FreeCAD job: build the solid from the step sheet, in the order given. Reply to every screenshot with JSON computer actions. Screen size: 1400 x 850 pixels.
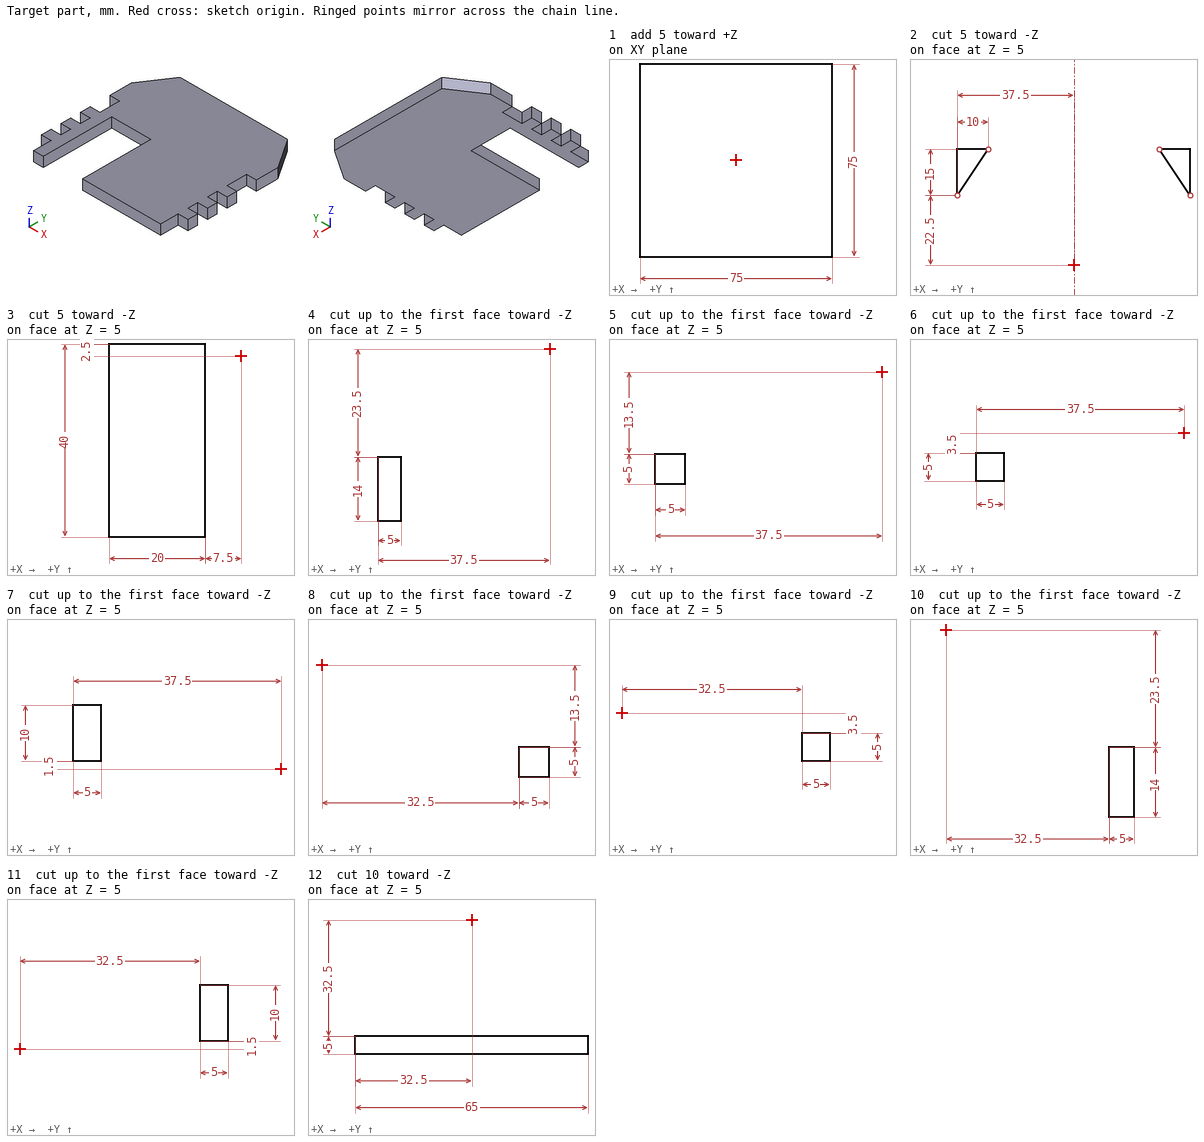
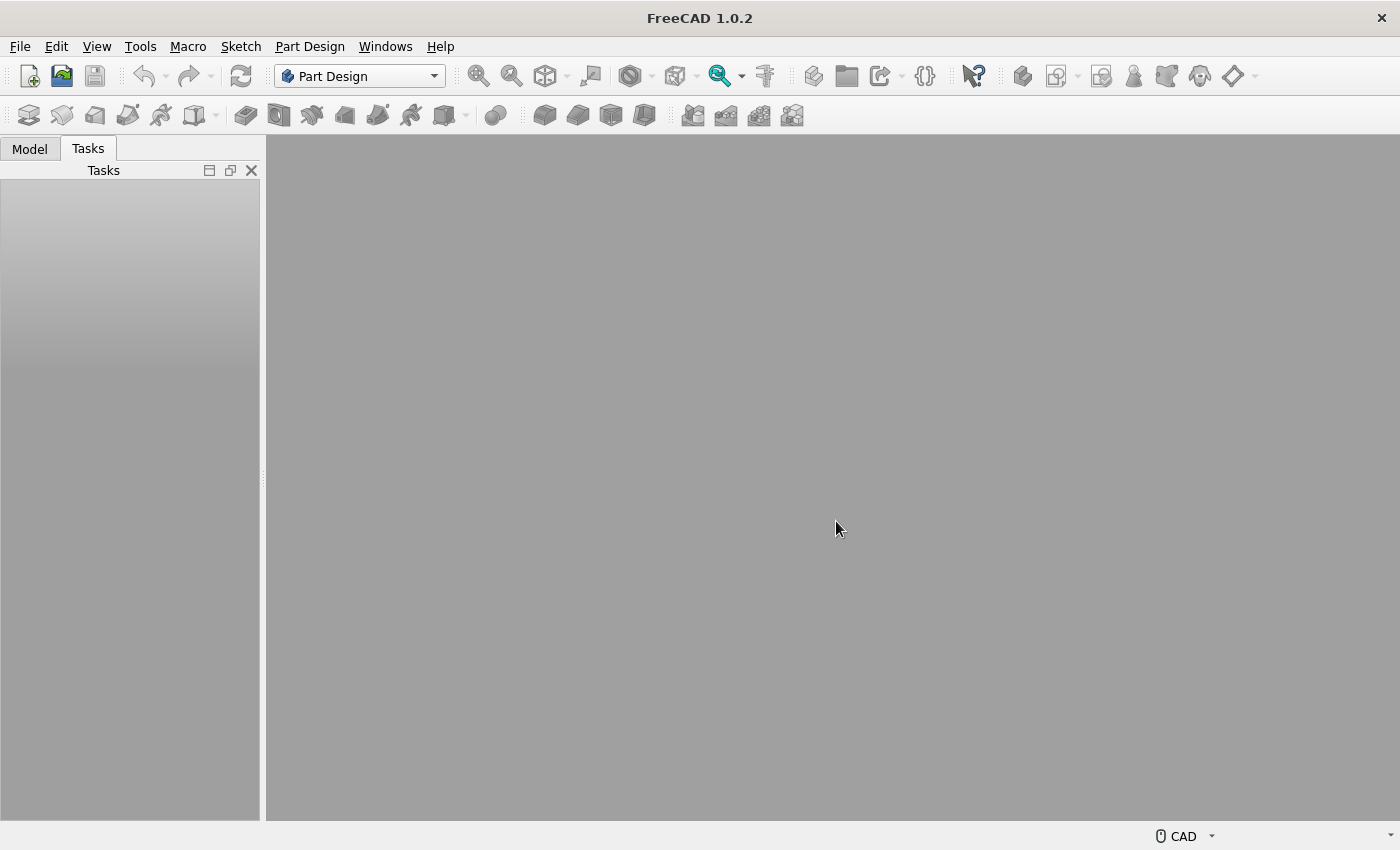
{"action": "left_click", "coordinate": [29, 76]}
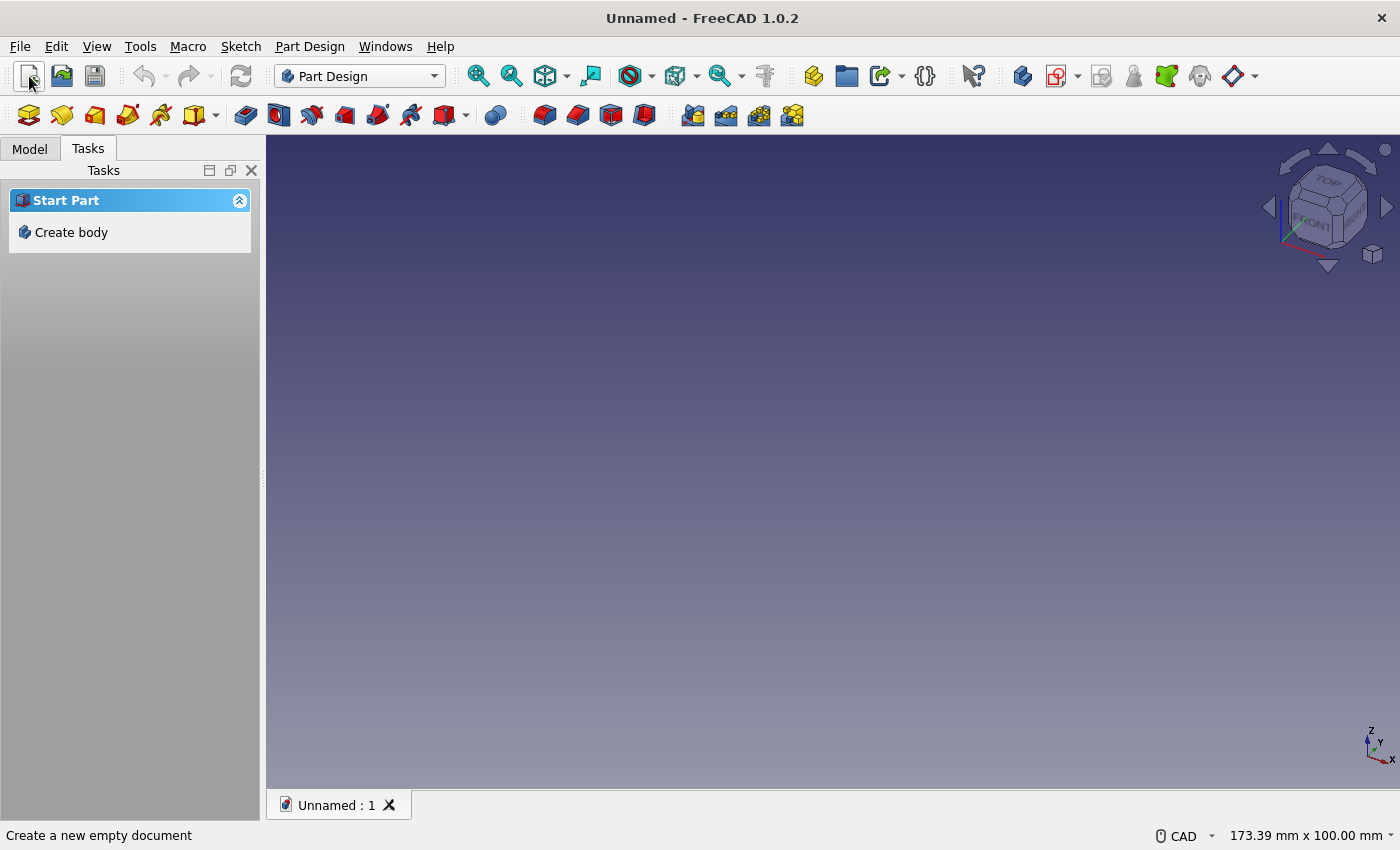
{"action": "left_click", "coordinate": [1056, 76]}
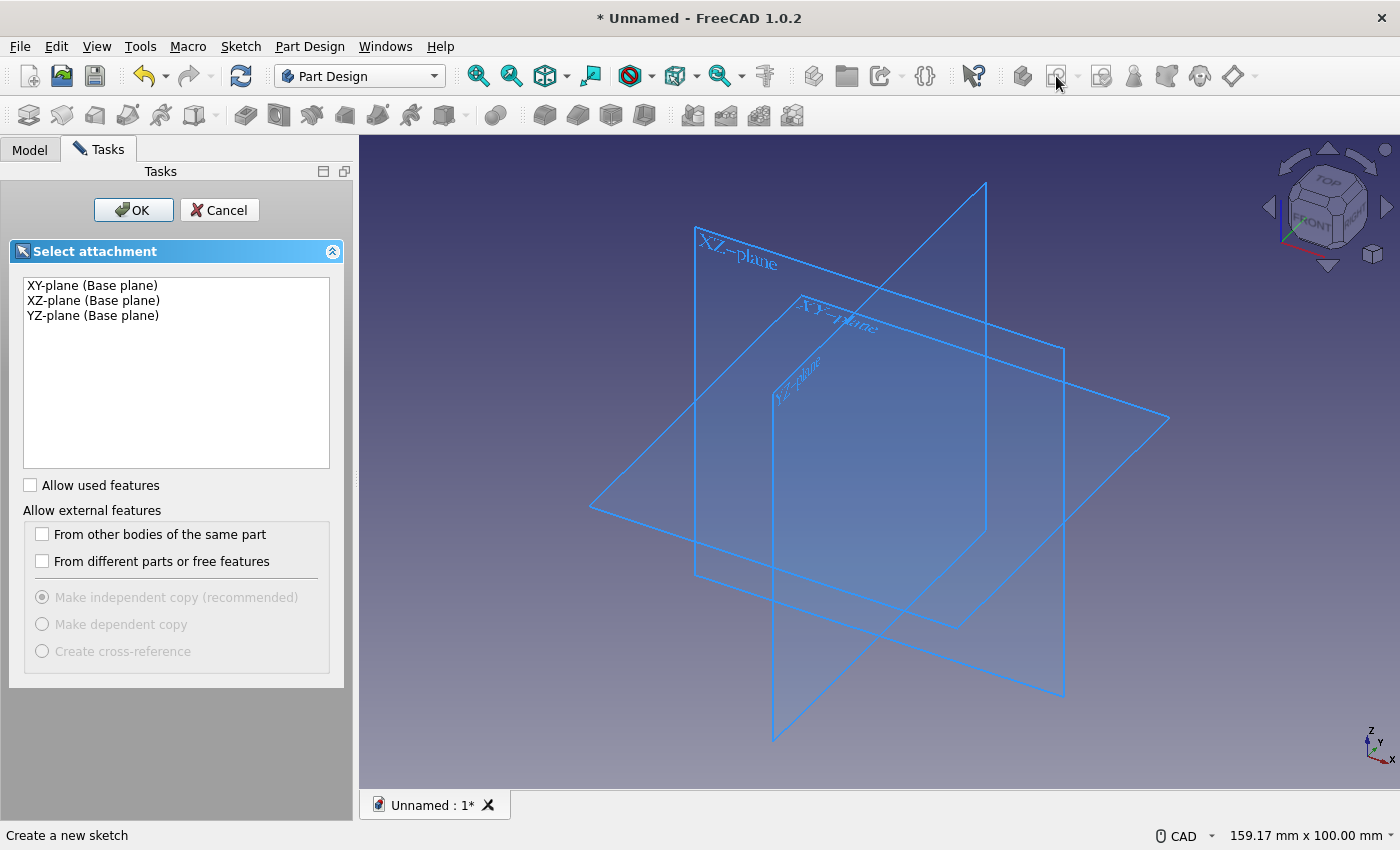
{"action": "left_click", "coordinate": [84, 286]}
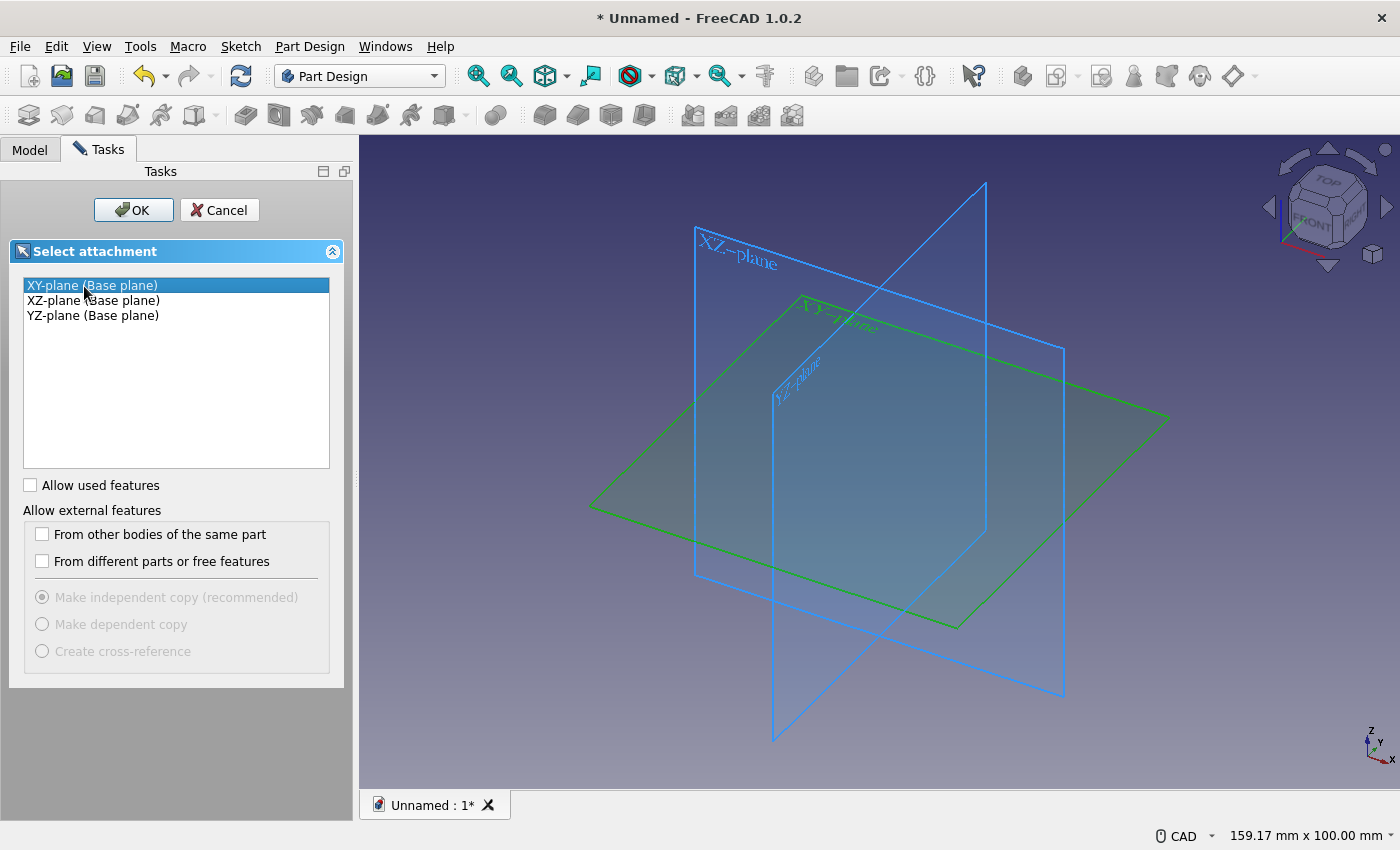
{"action": "left_click", "coordinate": [134, 210]}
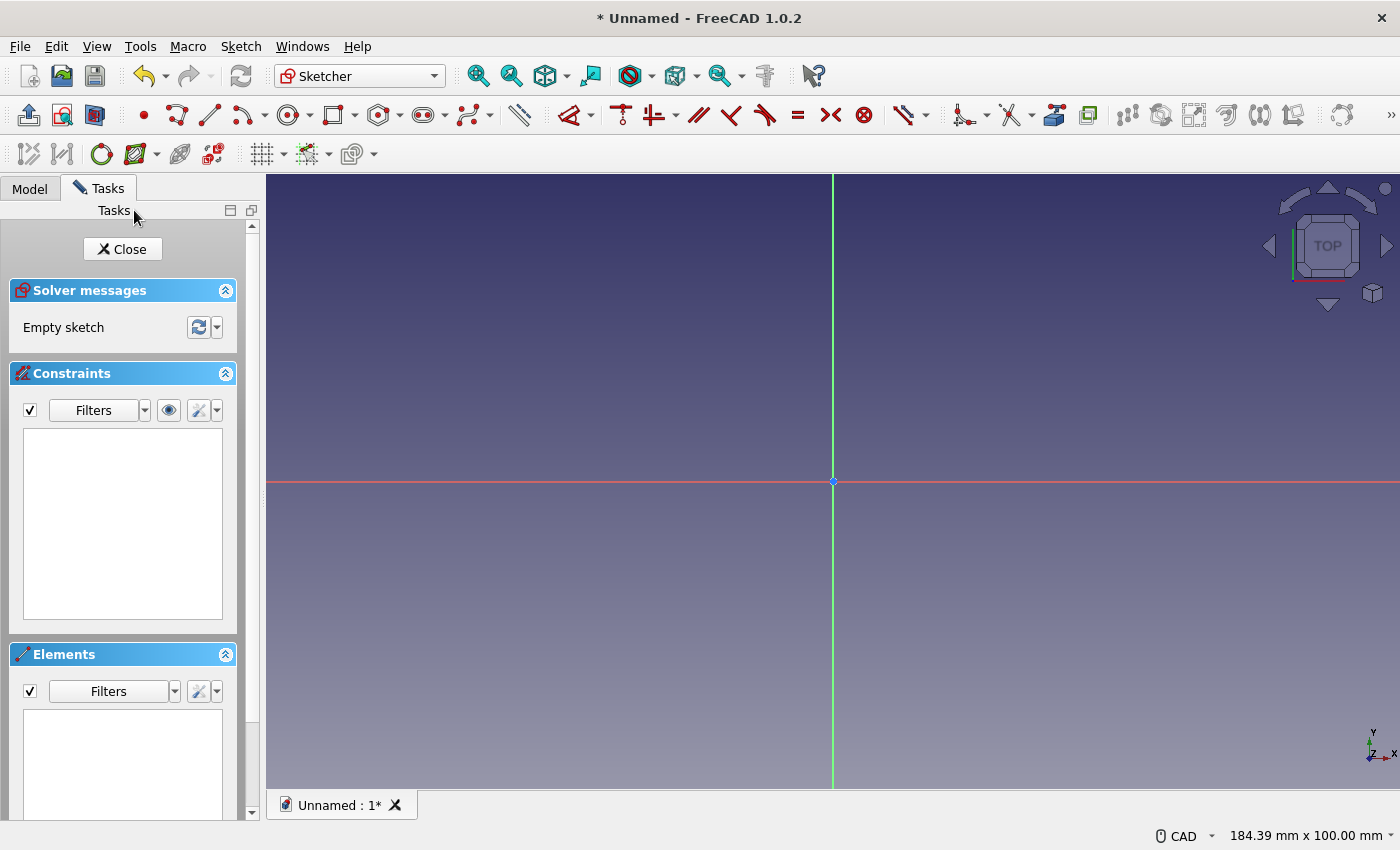
{"action": "key", "text": "g v"}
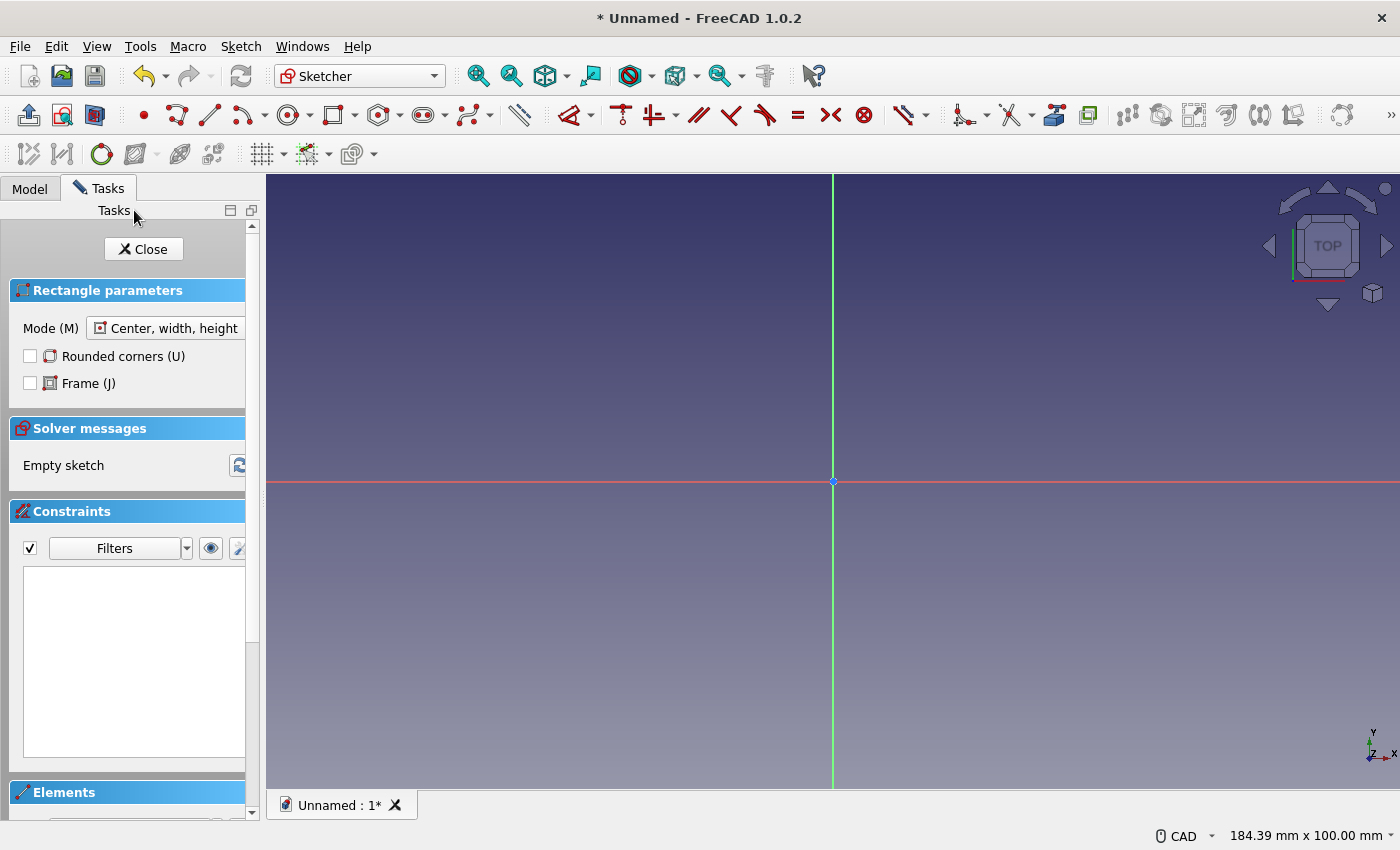
{"action": "left_click", "coordinate": [833, 482]}
{"action": "left_click", "coordinate": [1064, 251]}
{"action": "key", "text": "Escape"}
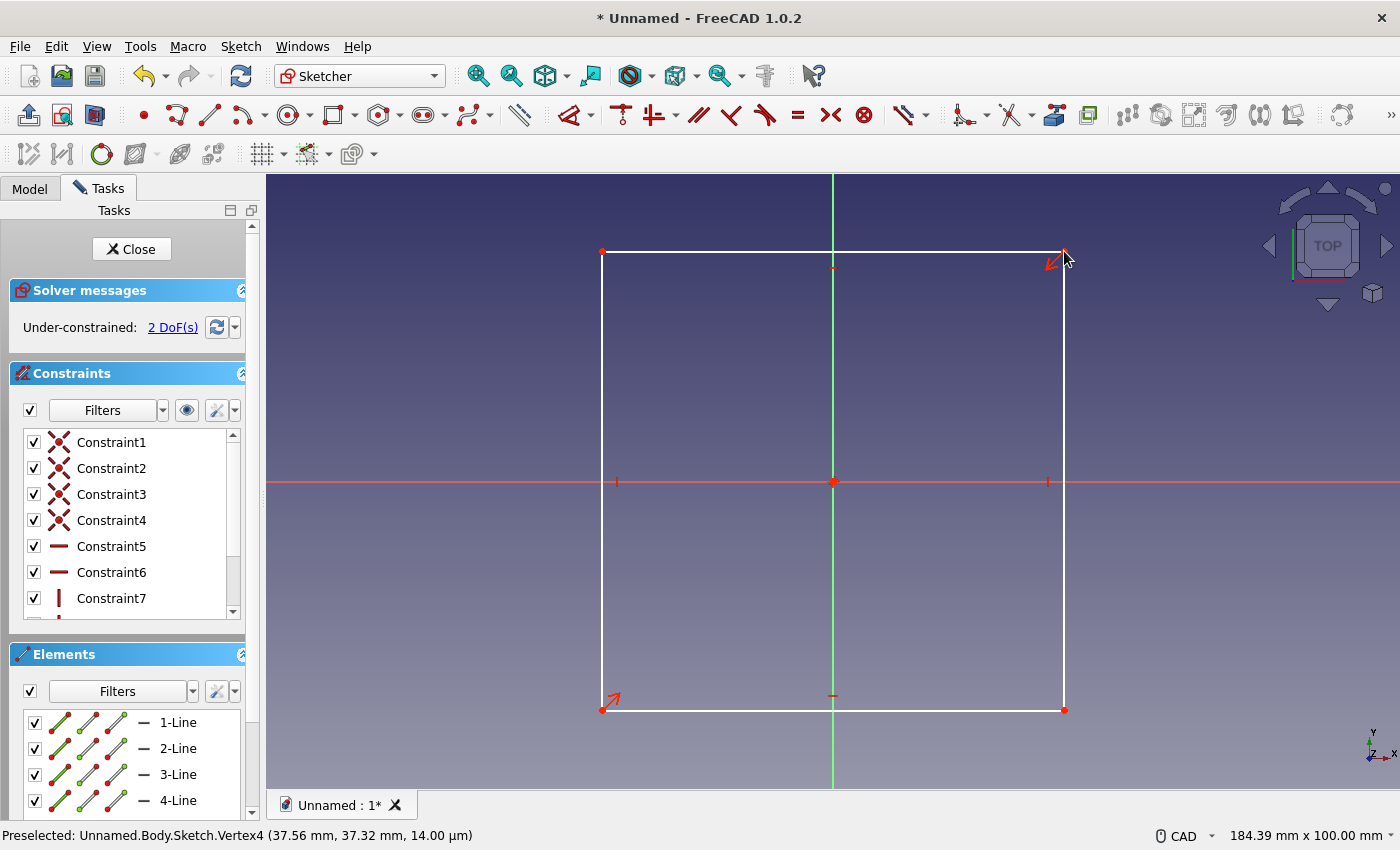
{"action": "left_click", "coordinate": [568, 116]}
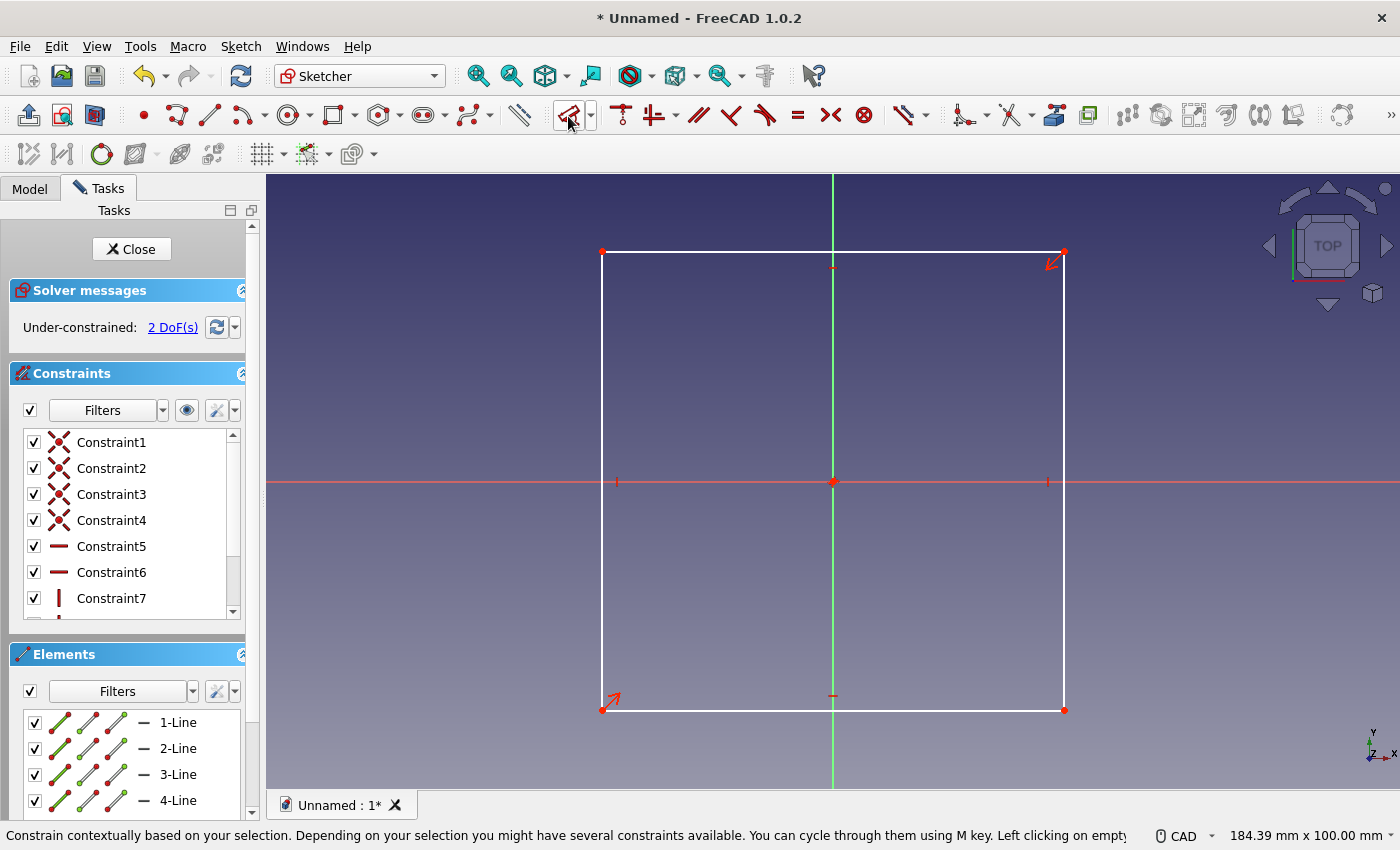
{"action": "left_click", "coordinate": [741, 711]}
{"action": "left_click", "coordinate": [727, 745]}